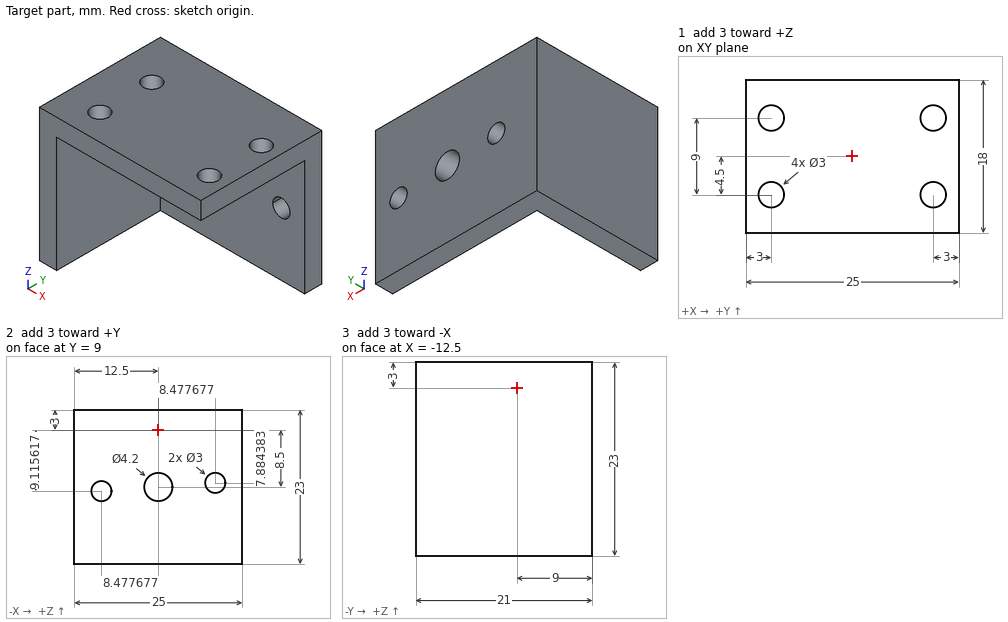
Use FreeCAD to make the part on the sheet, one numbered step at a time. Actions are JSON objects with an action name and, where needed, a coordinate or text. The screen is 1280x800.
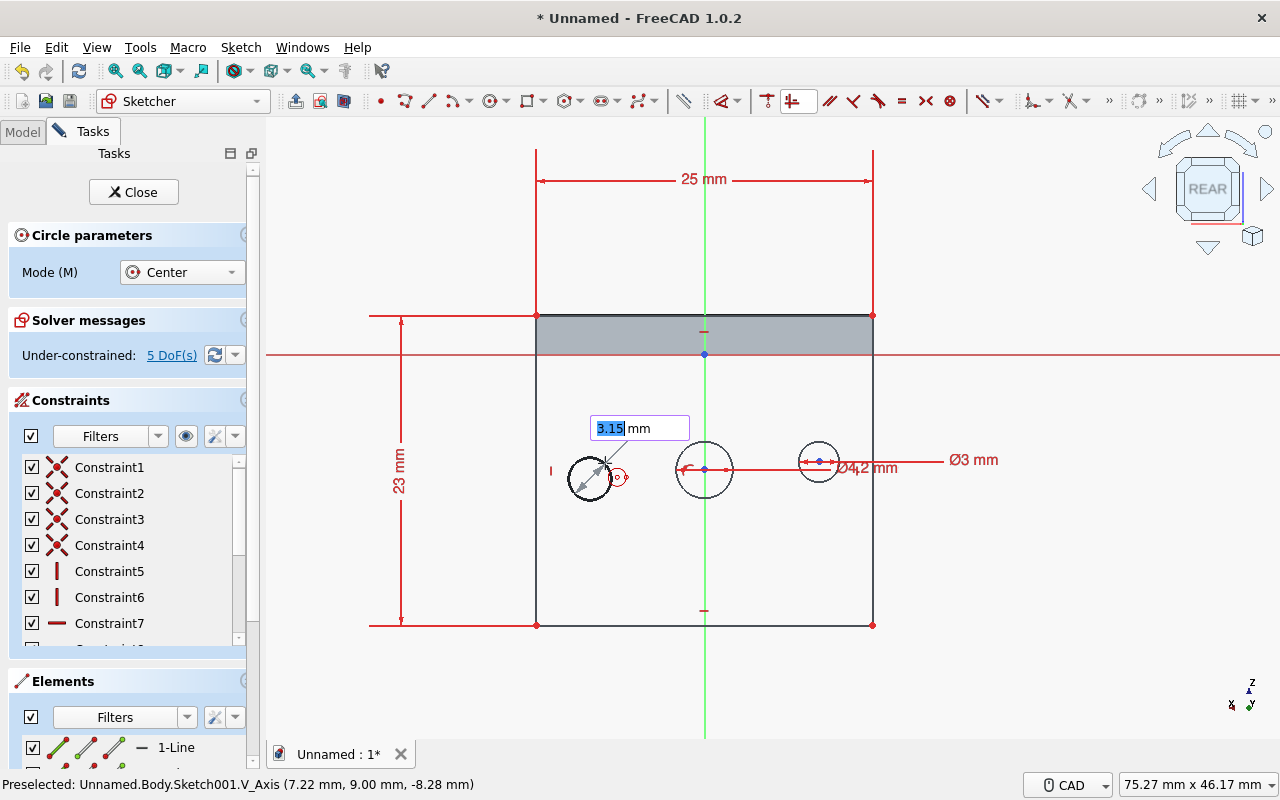
{"action": "type", "text": "3"}
{"action": "key", "text": "Return"}
{"action": "key", "text": "Escape"}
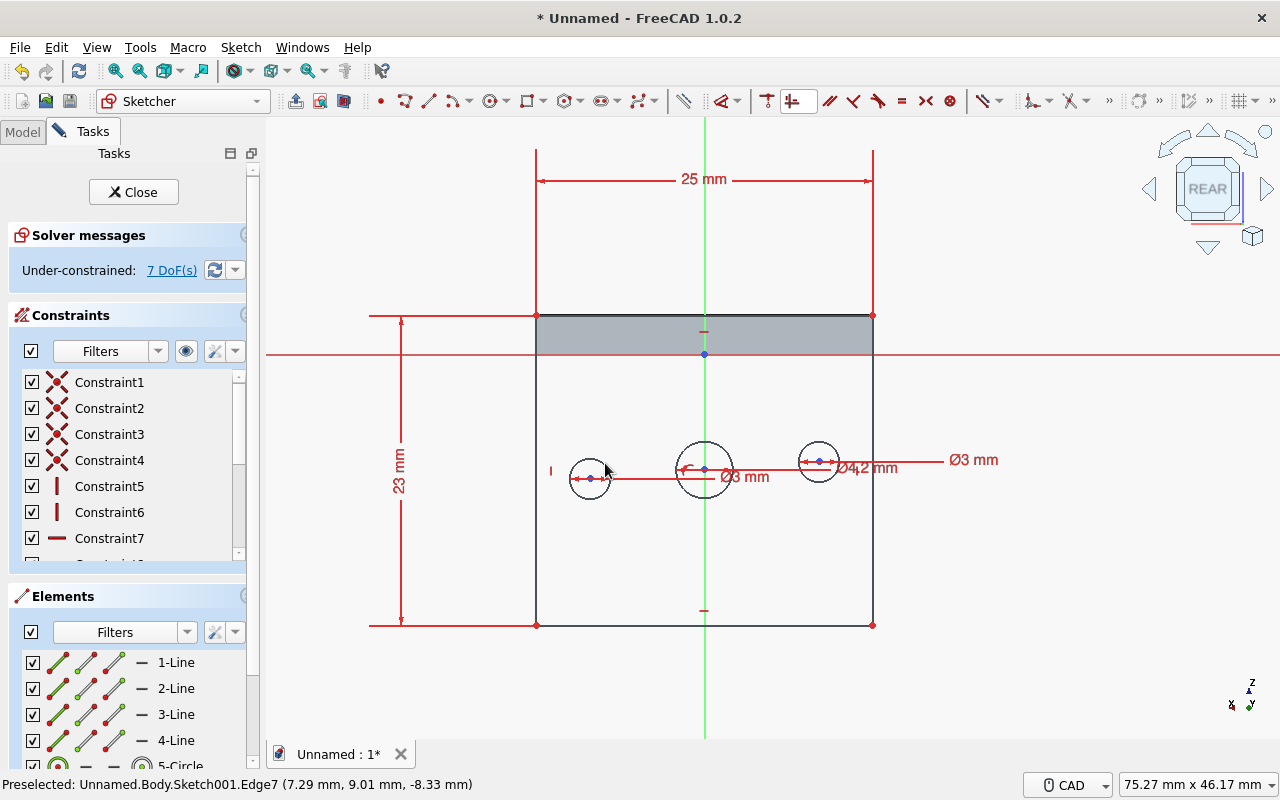
{"action": "key", "text": "d"}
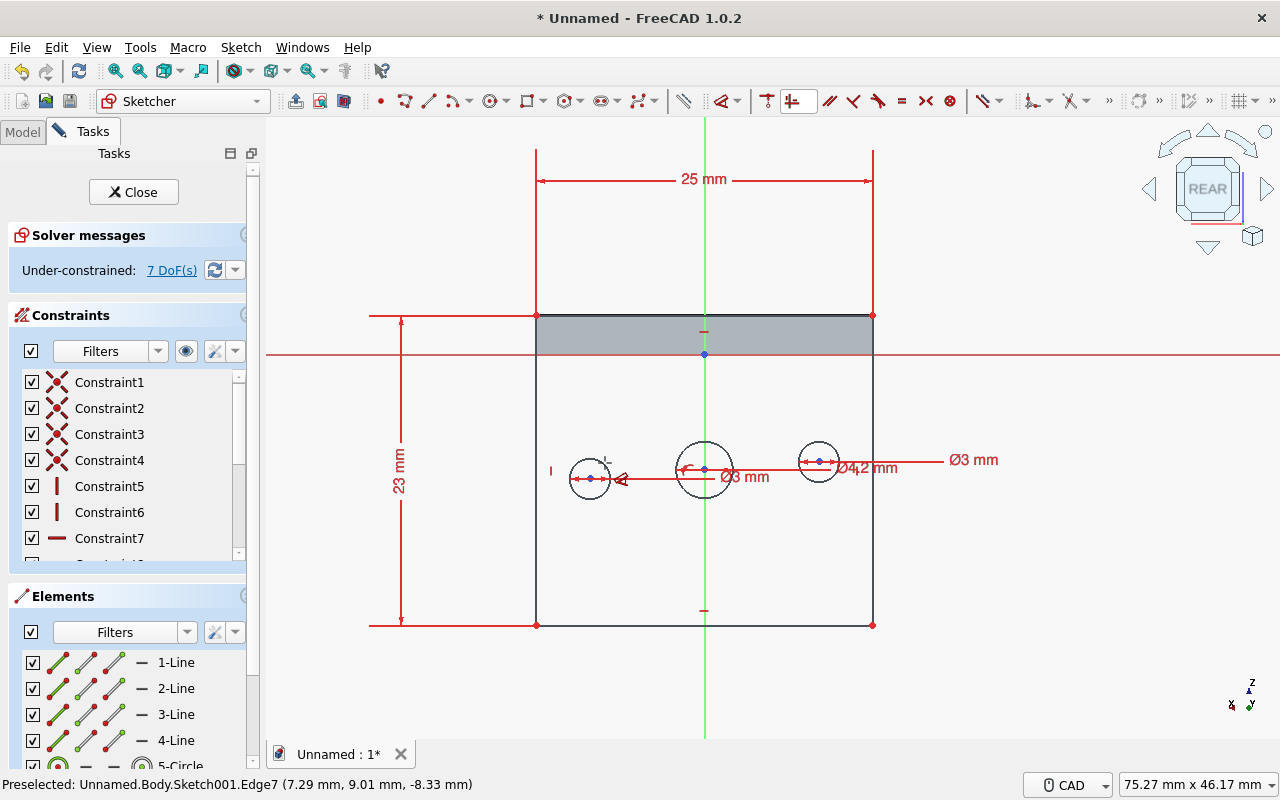
{"action": "left_click", "coordinate": [536, 316]}
{"action": "left_click", "coordinate": [502, 335]}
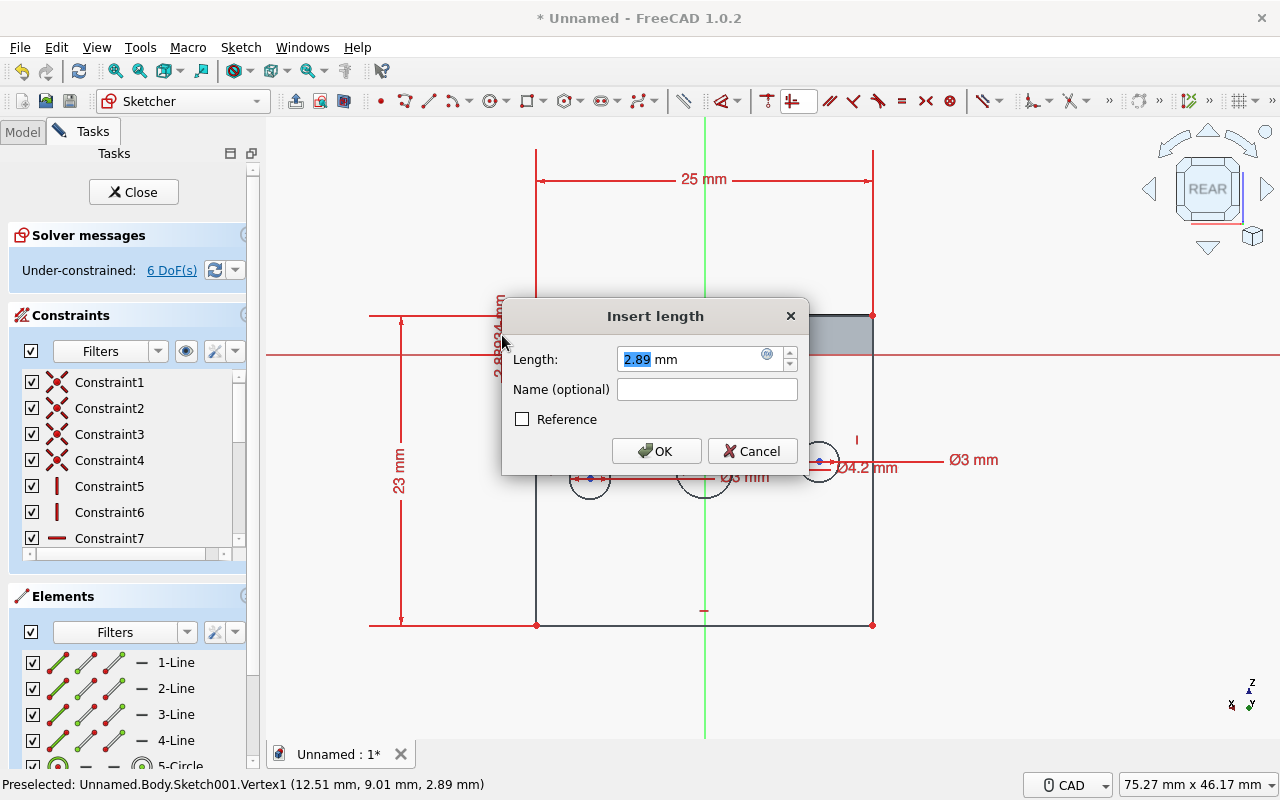
{"action": "type", "text": "3"}
{"action": "key", "text": "Return"}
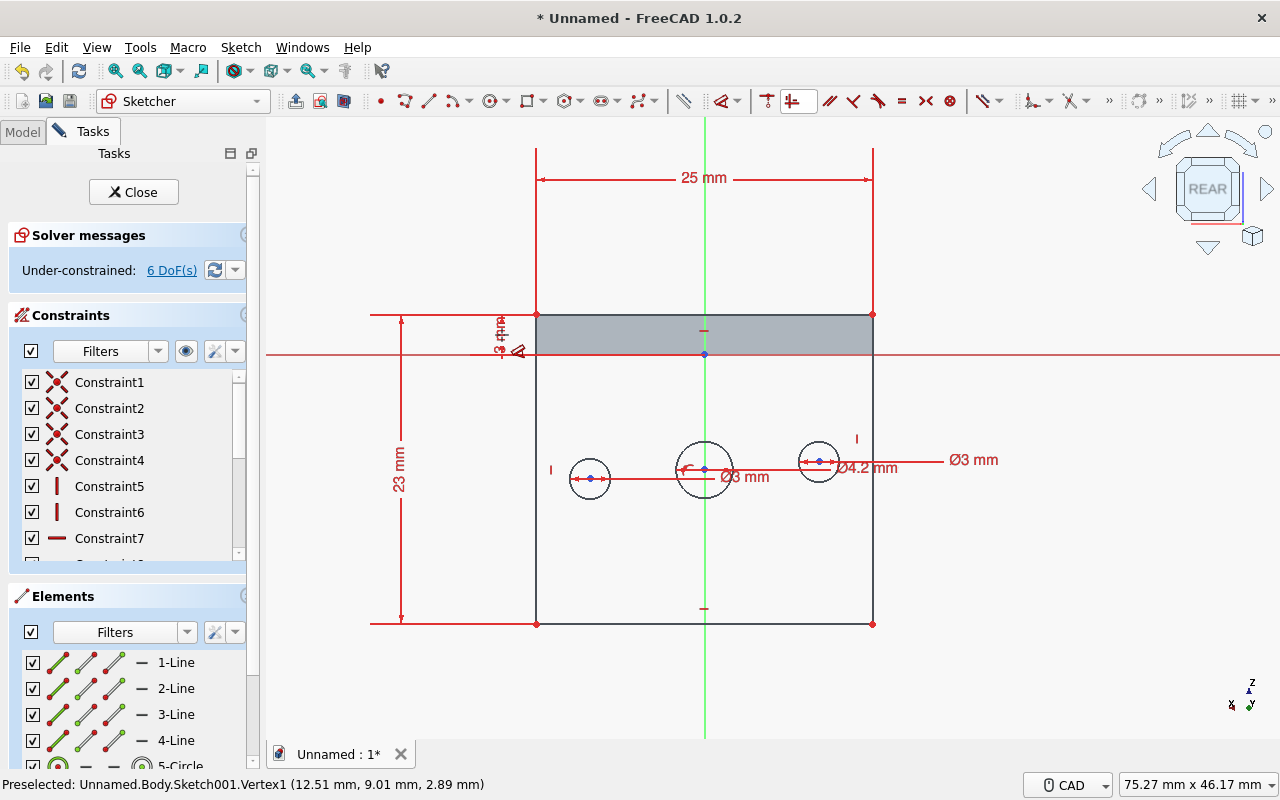
{"action": "left_click", "coordinate": [705, 470]}
{"action": "left_click", "coordinate": [739, 412]}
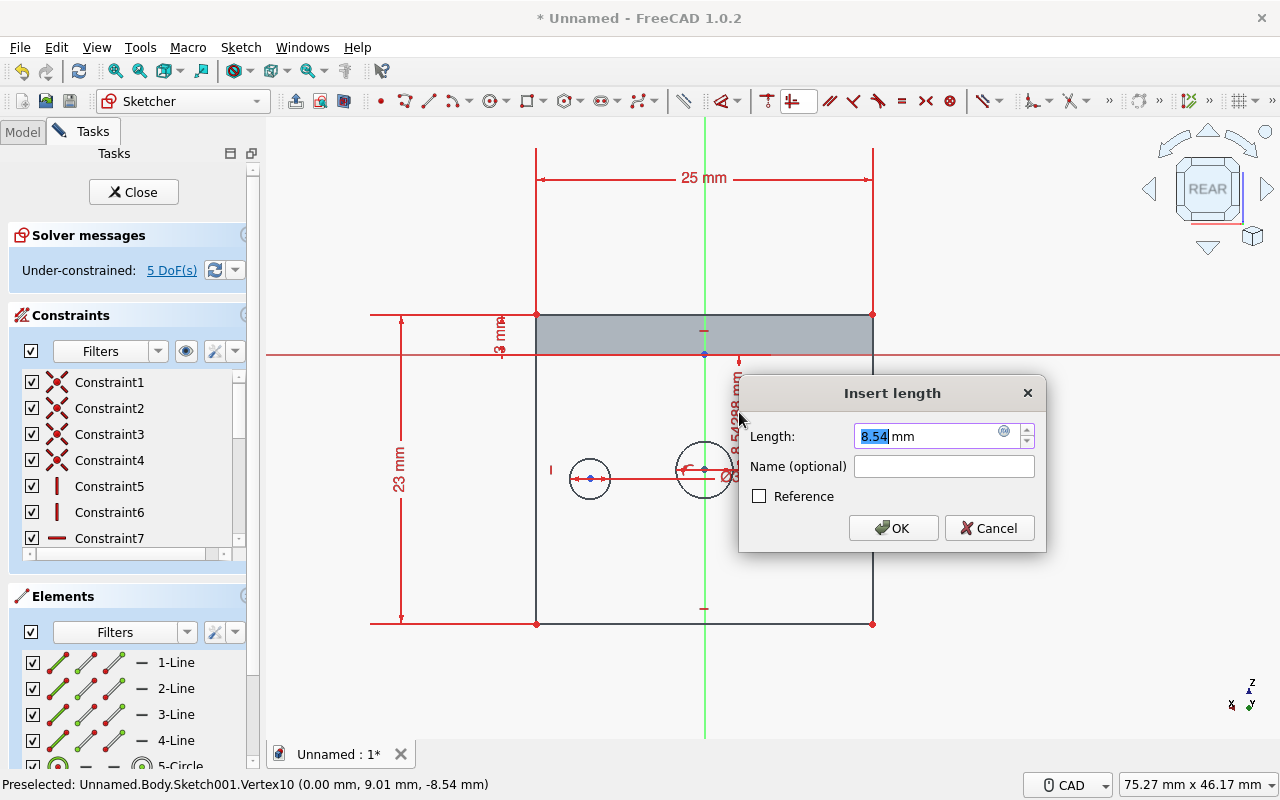
{"action": "type", "text": "8.5"}
{"action": "key", "text": "Return"}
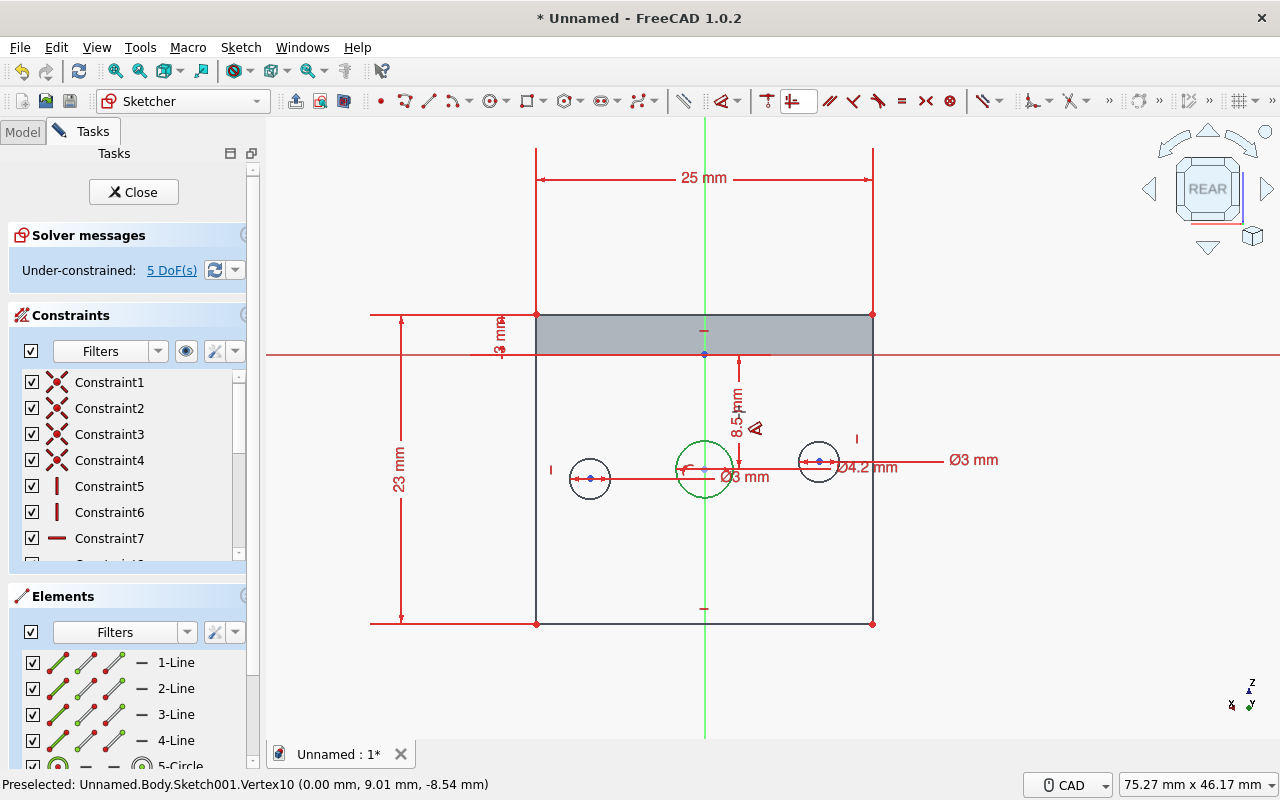
{"action": "left_click", "coordinate": [536, 315]}
{"action": "left_click", "coordinate": [620, 281]}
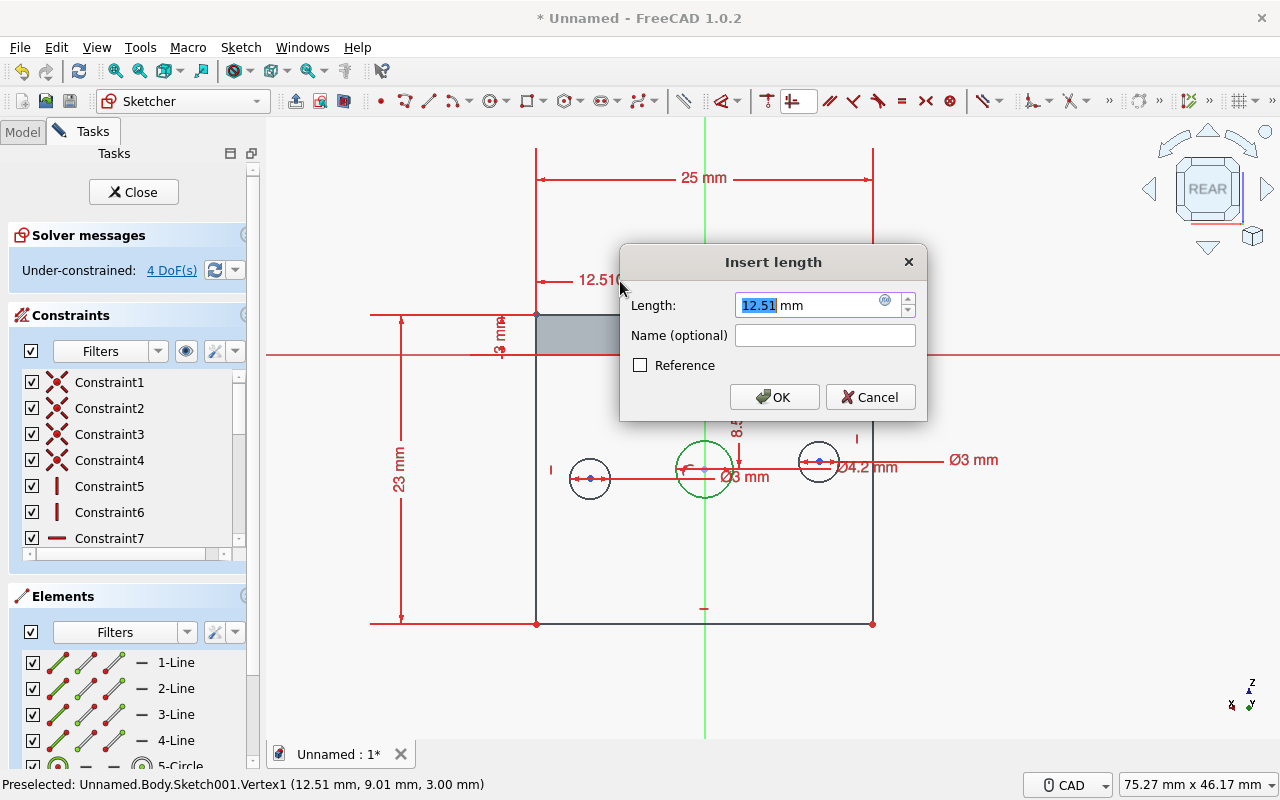
{"action": "type", "text": "12.5"}
{"action": "key", "text": "Return"}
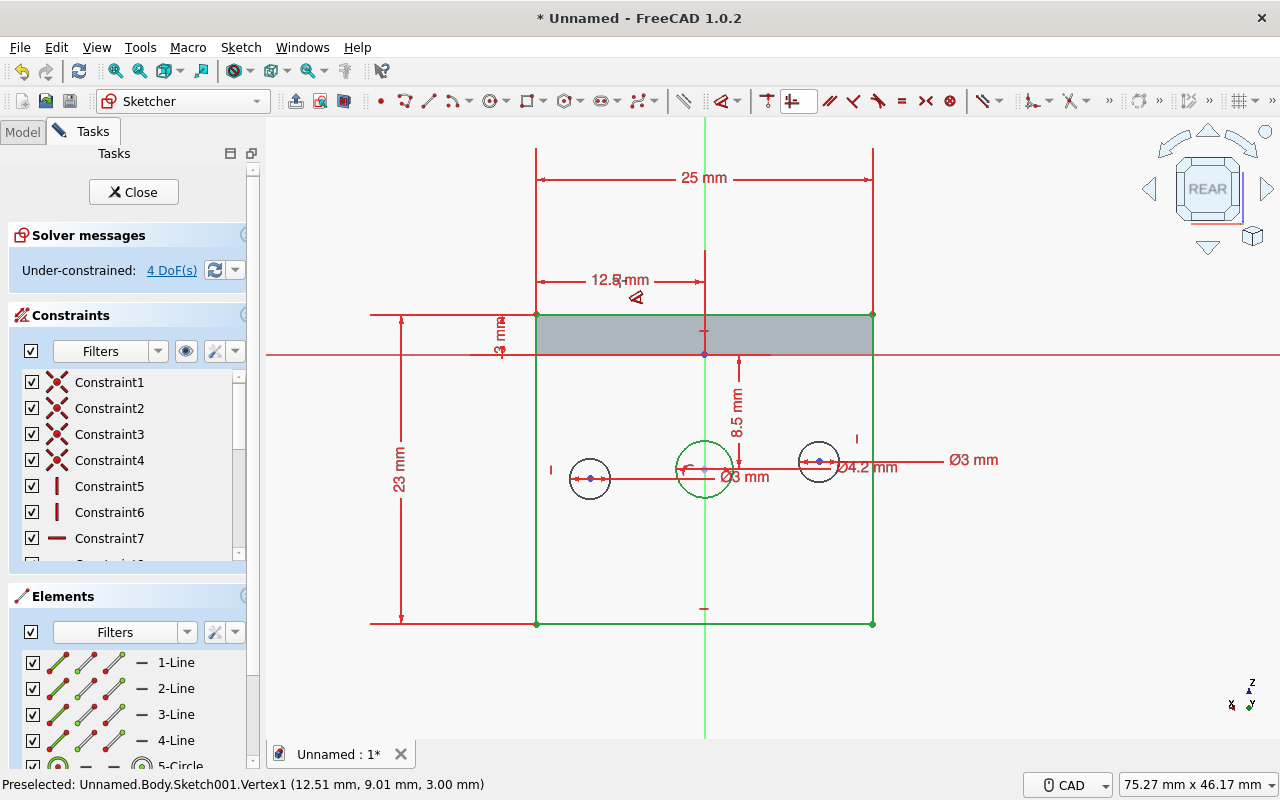
{"action": "left_click", "coordinate": [819, 462]}
{"action": "left_click", "coordinate": [762, 496]}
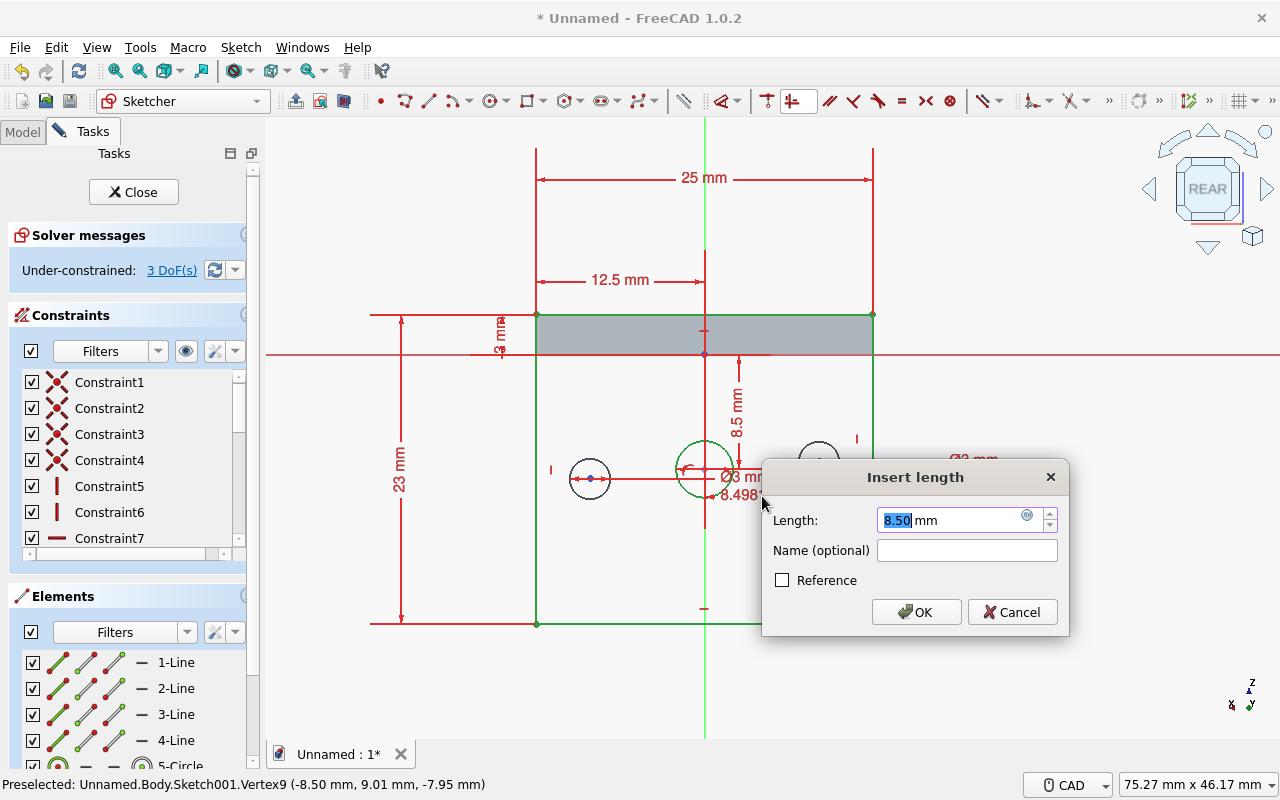
{"action": "type", "text": "8.477677"}
{"action": "key", "text": "Return"}